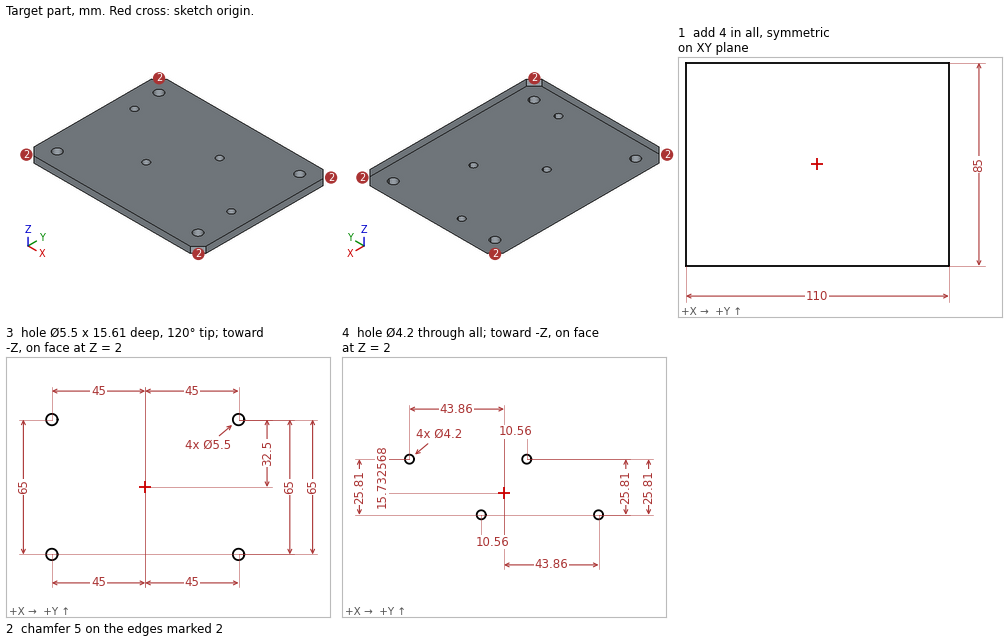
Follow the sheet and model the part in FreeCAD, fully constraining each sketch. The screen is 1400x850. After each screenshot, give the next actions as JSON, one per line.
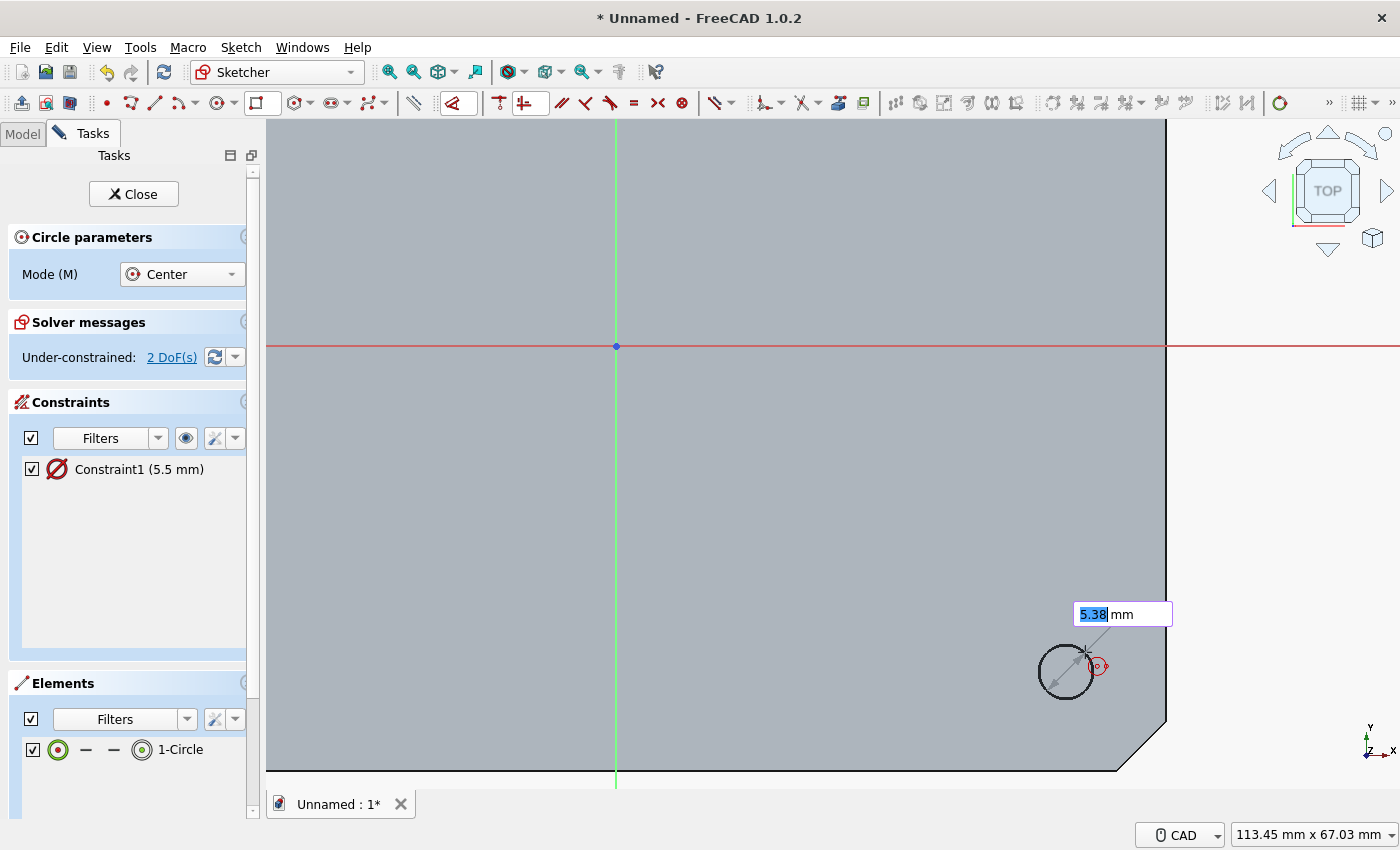
{"action": "type", "text": "5.5"}
{"action": "key", "text": "Return"}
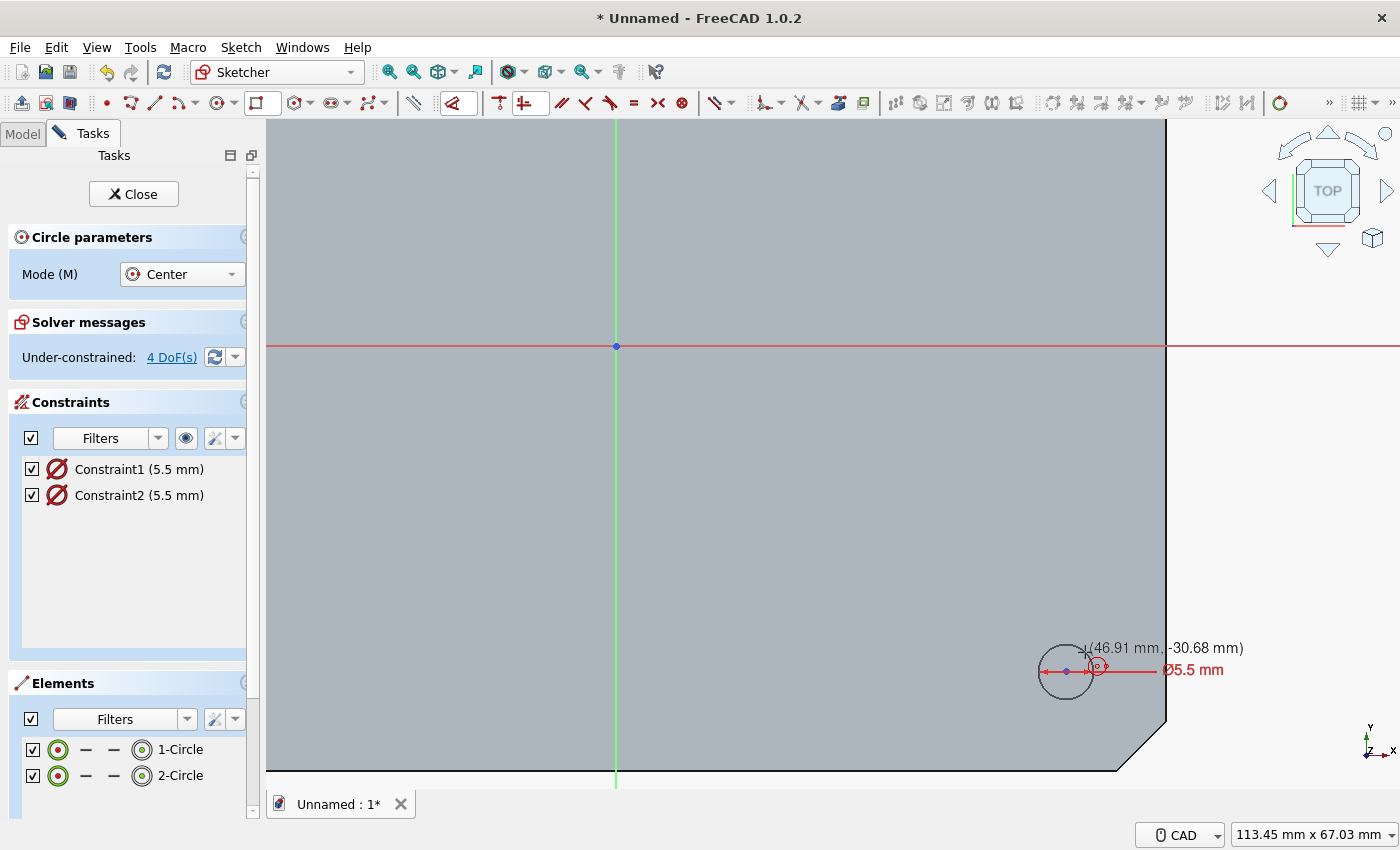
{"action": "scroll", "coordinate": [1066, 673], "scroll_direction": "down", "scroll_amount": 2}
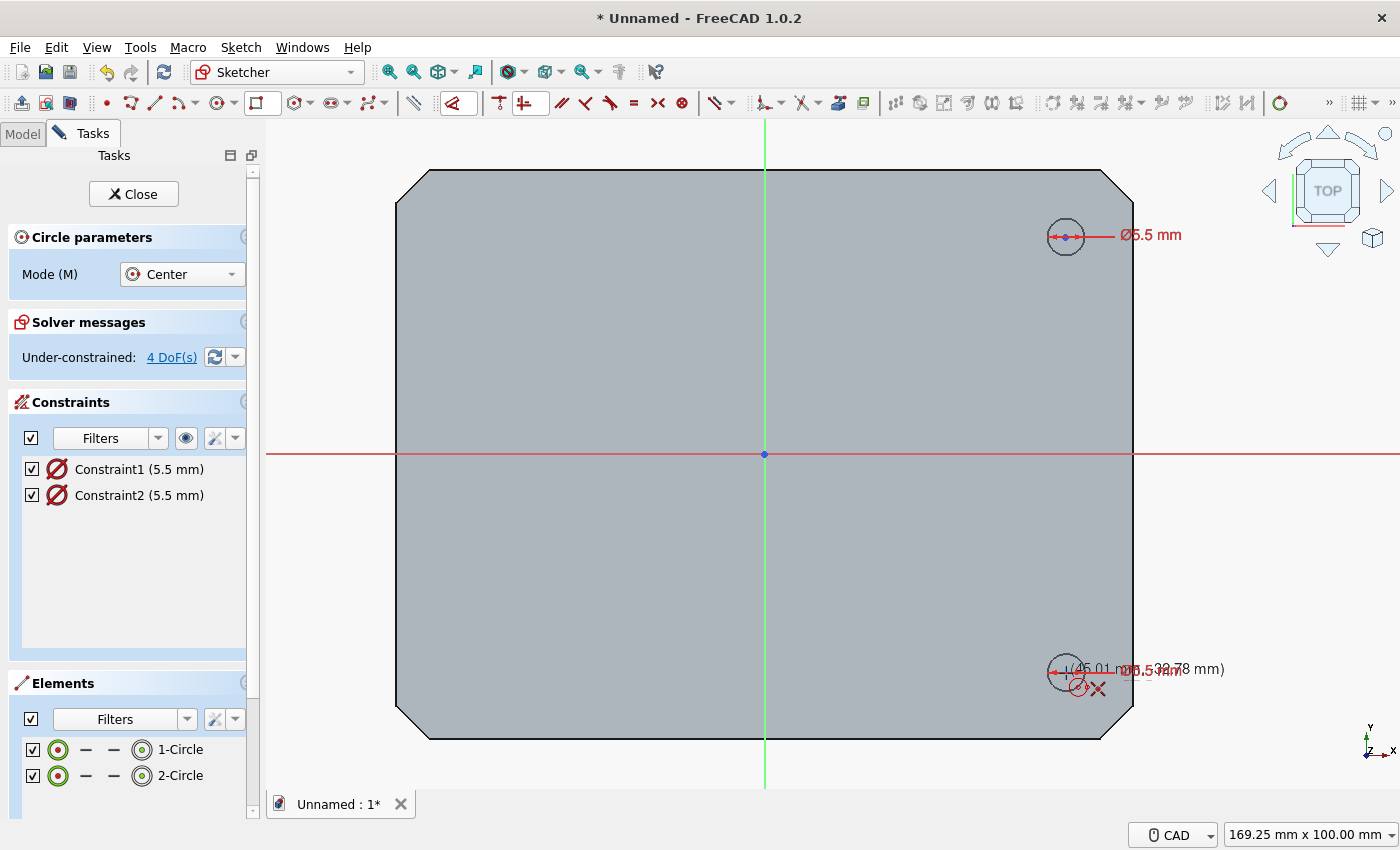
{"action": "scroll", "coordinate": [463, 672], "scroll_direction": "up", "scroll_amount": 2}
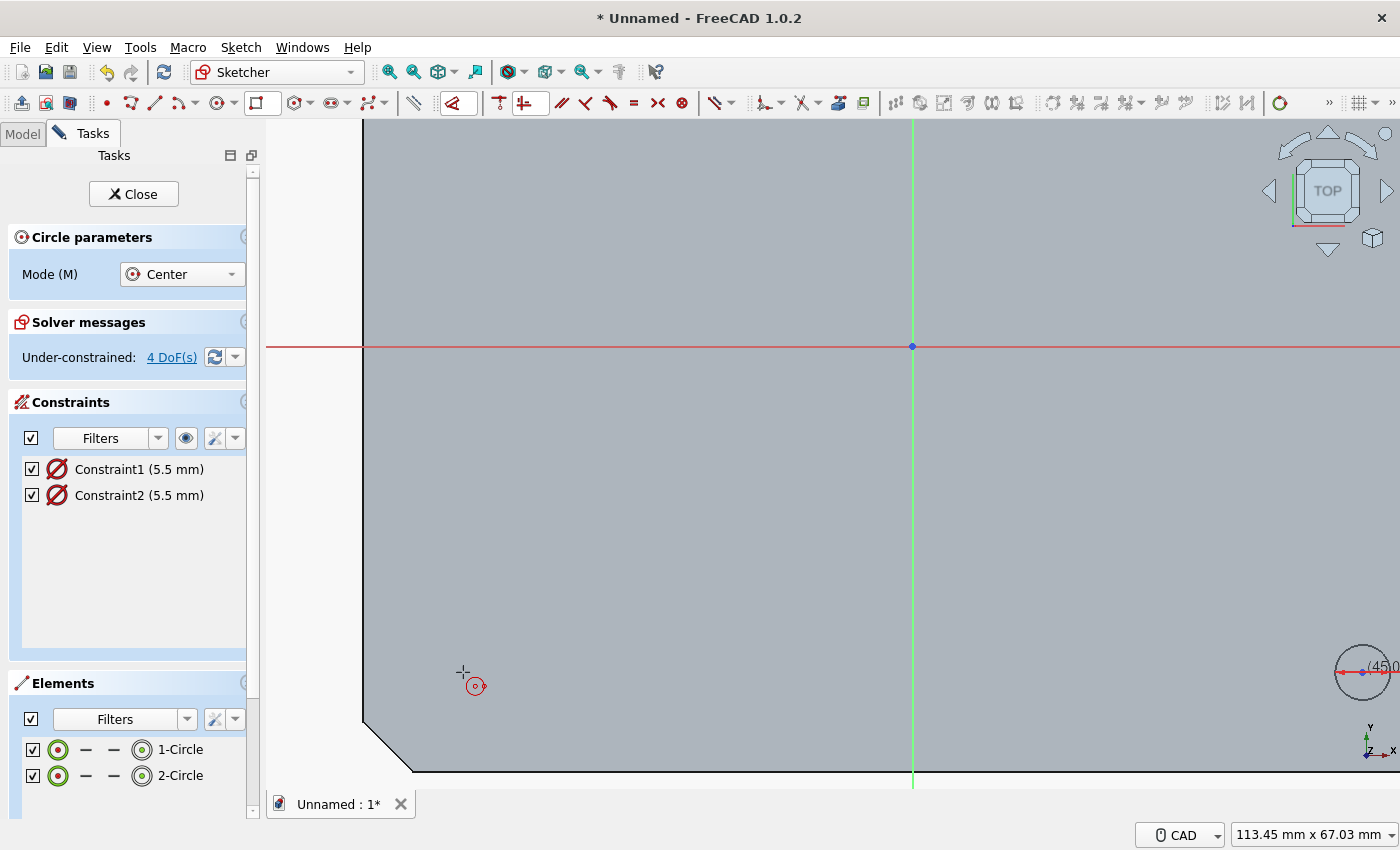
{"action": "left_click", "coordinate": [463, 672]}
{"action": "mouse_move", "coordinate": [483, 652]}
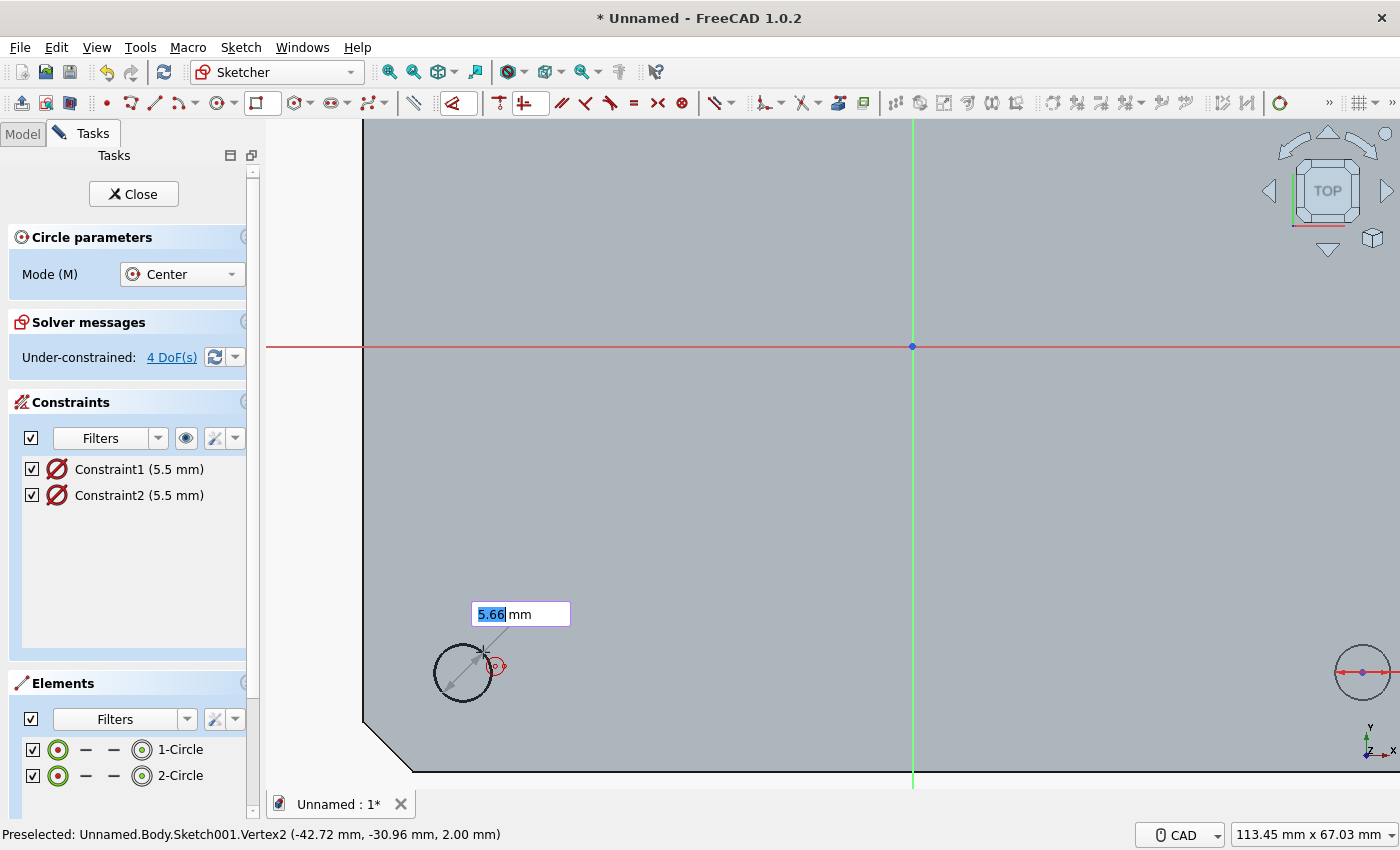
{"action": "type", "text": "5.5"}
{"action": "key", "text": "Return"}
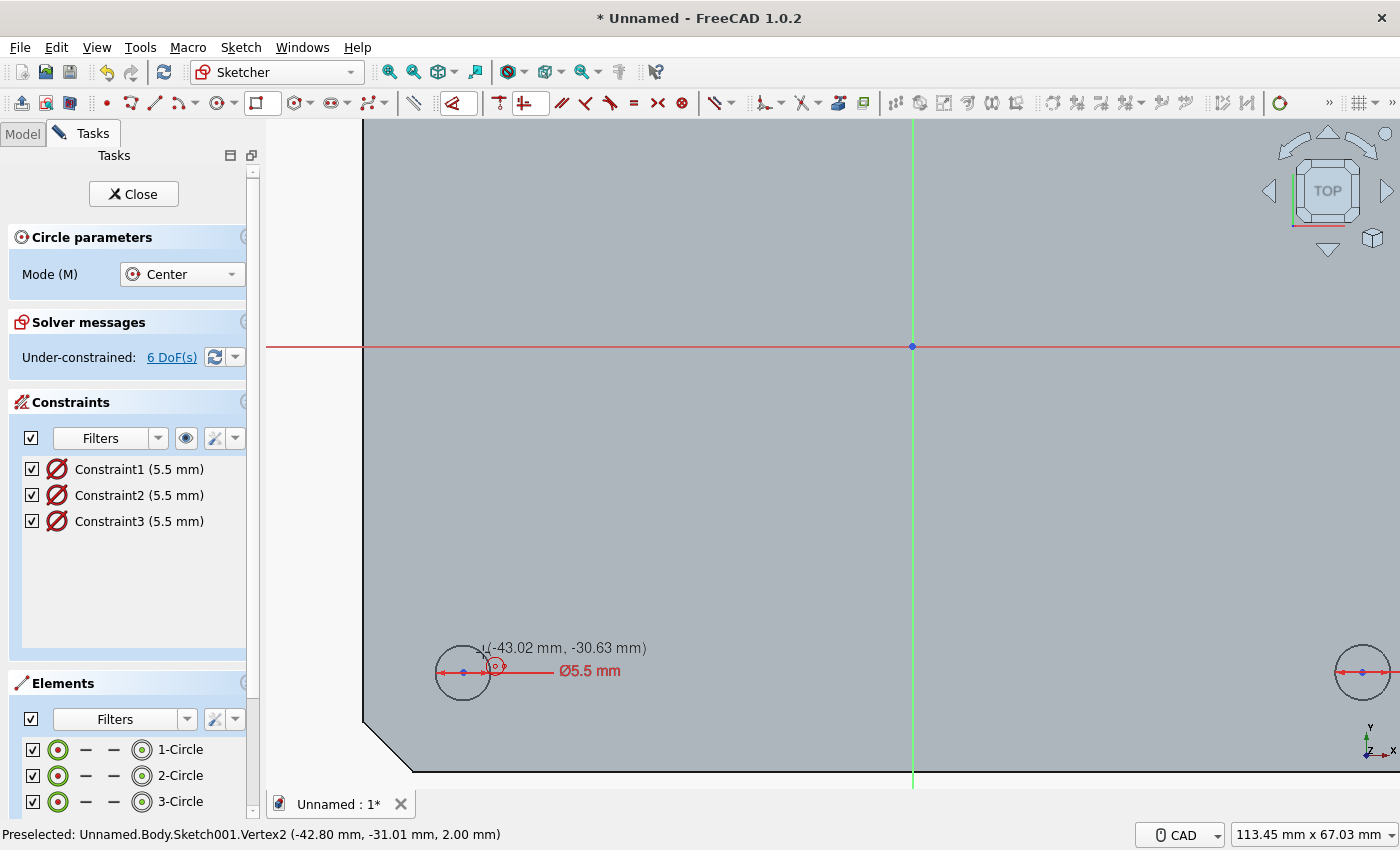
{"action": "scroll", "coordinate": [463, 672], "scroll_direction": "down", "scroll_amount": 2}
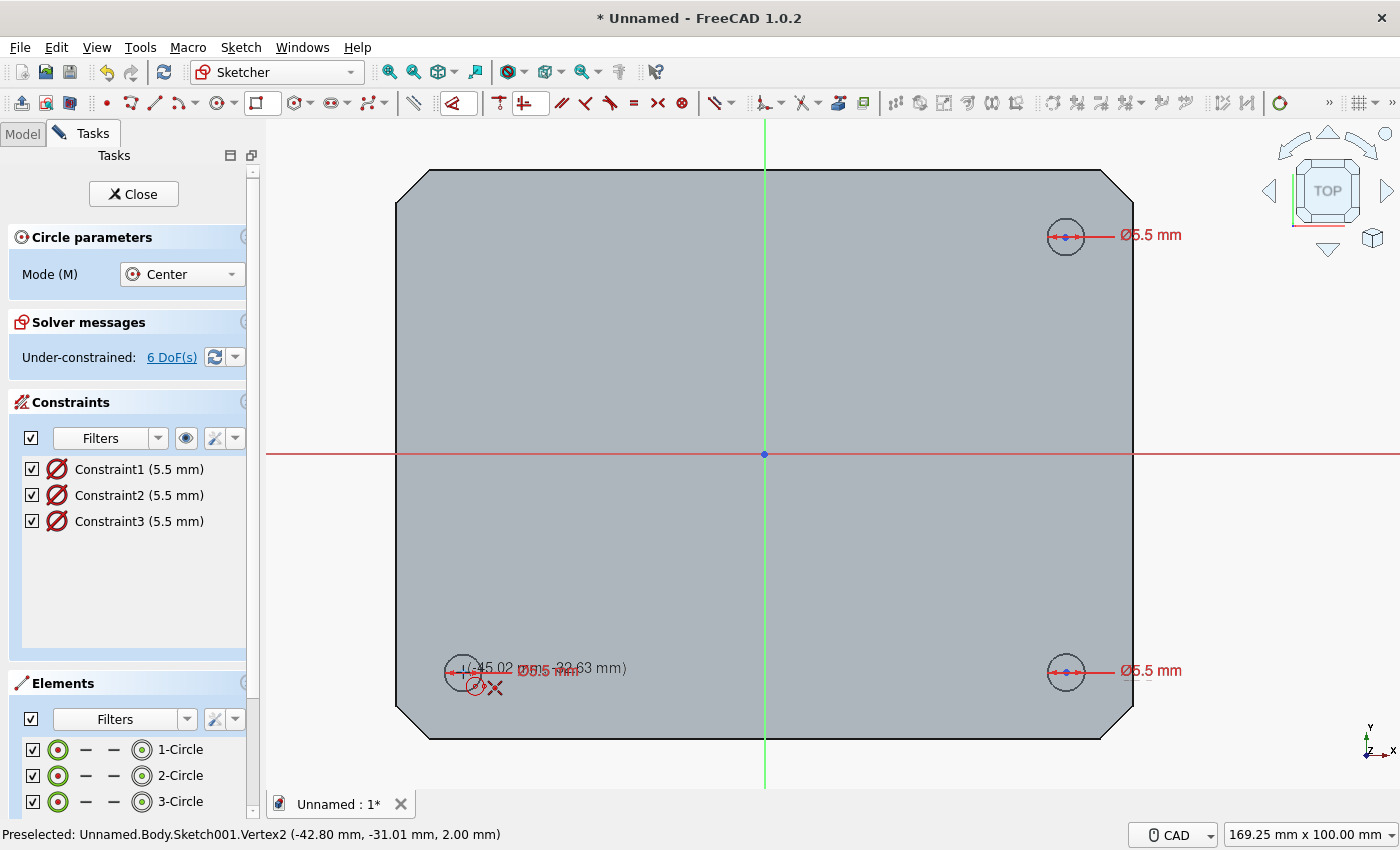
{"action": "scroll", "coordinate": [463, 237], "scroll_direction": "up", "scroll_amount": 2}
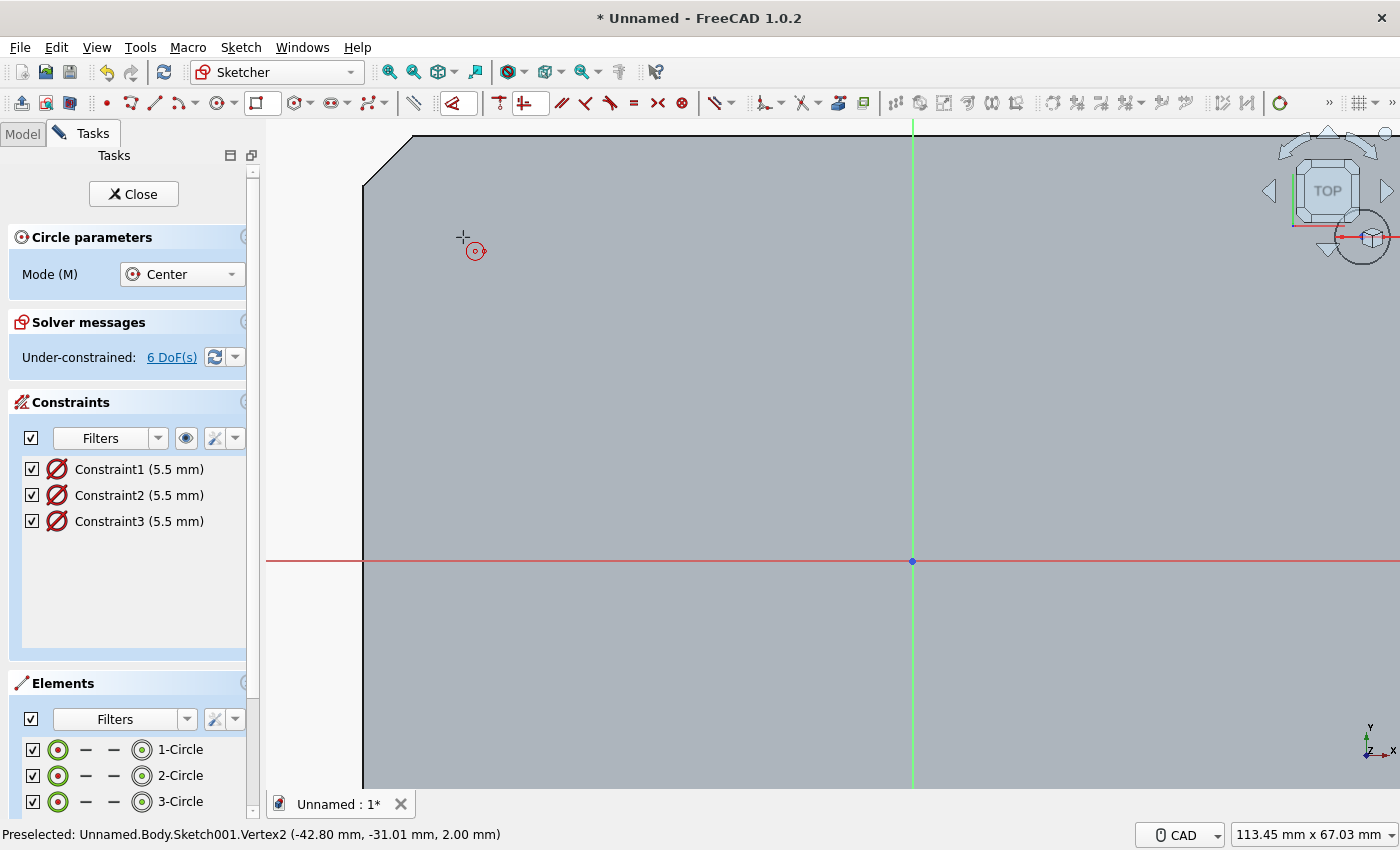
{"action": "left_click", "coordinate": [463, 236]}
{"action": "mouse_move", "coordinate": [483, 217]}